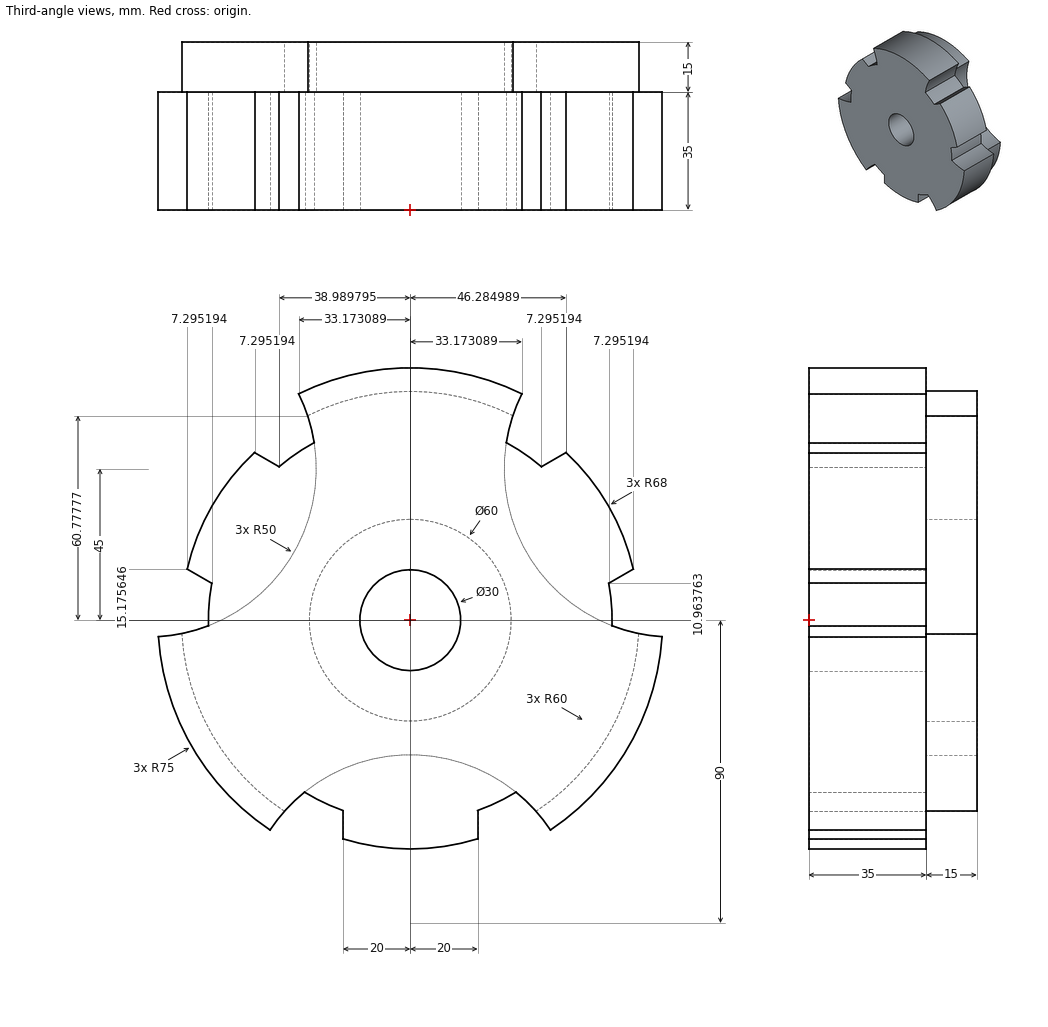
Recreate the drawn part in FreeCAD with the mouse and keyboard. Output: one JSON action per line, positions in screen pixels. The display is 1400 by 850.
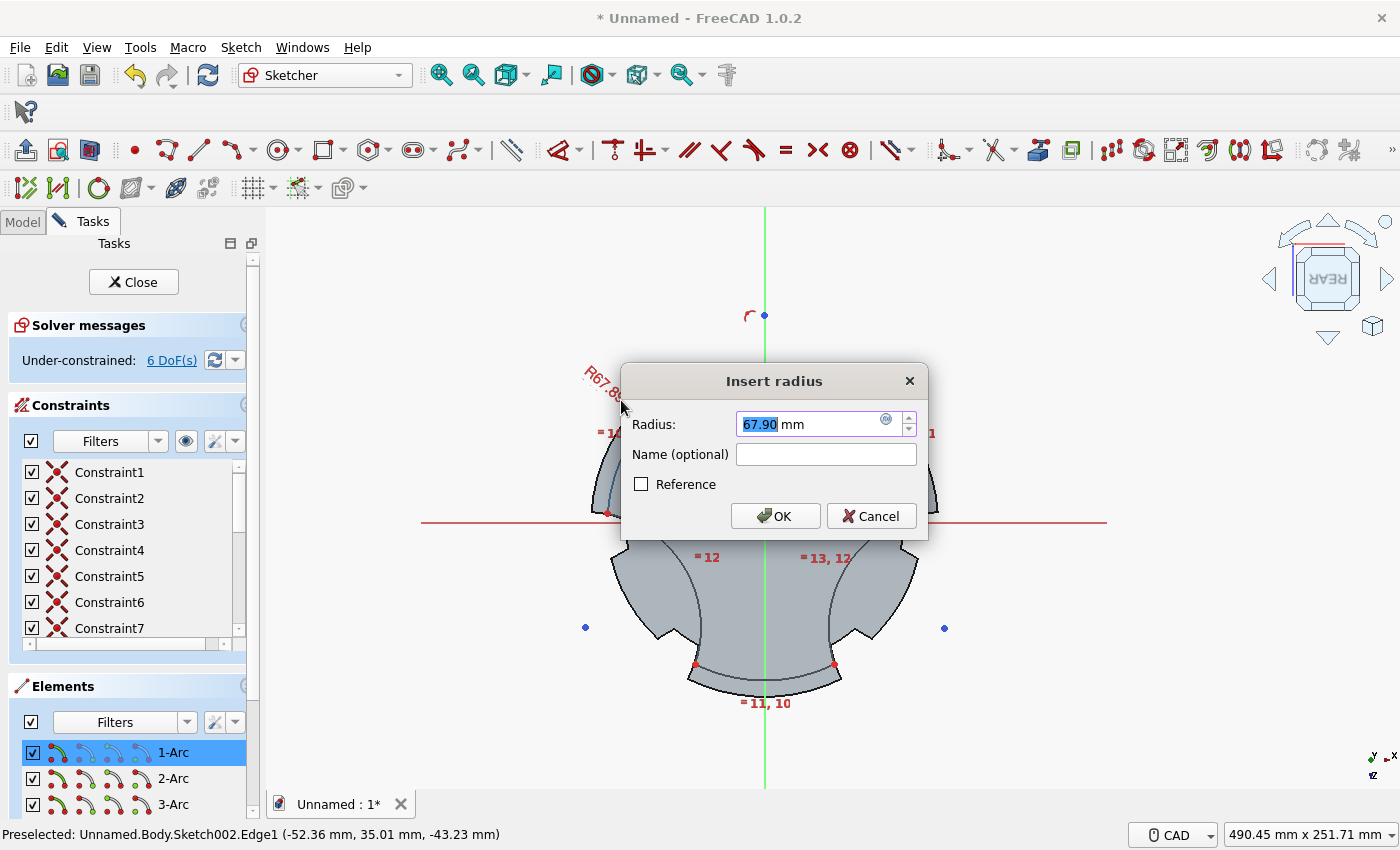
{"action": "type", "text": "68"}
{"action": "key", "text": "Return"}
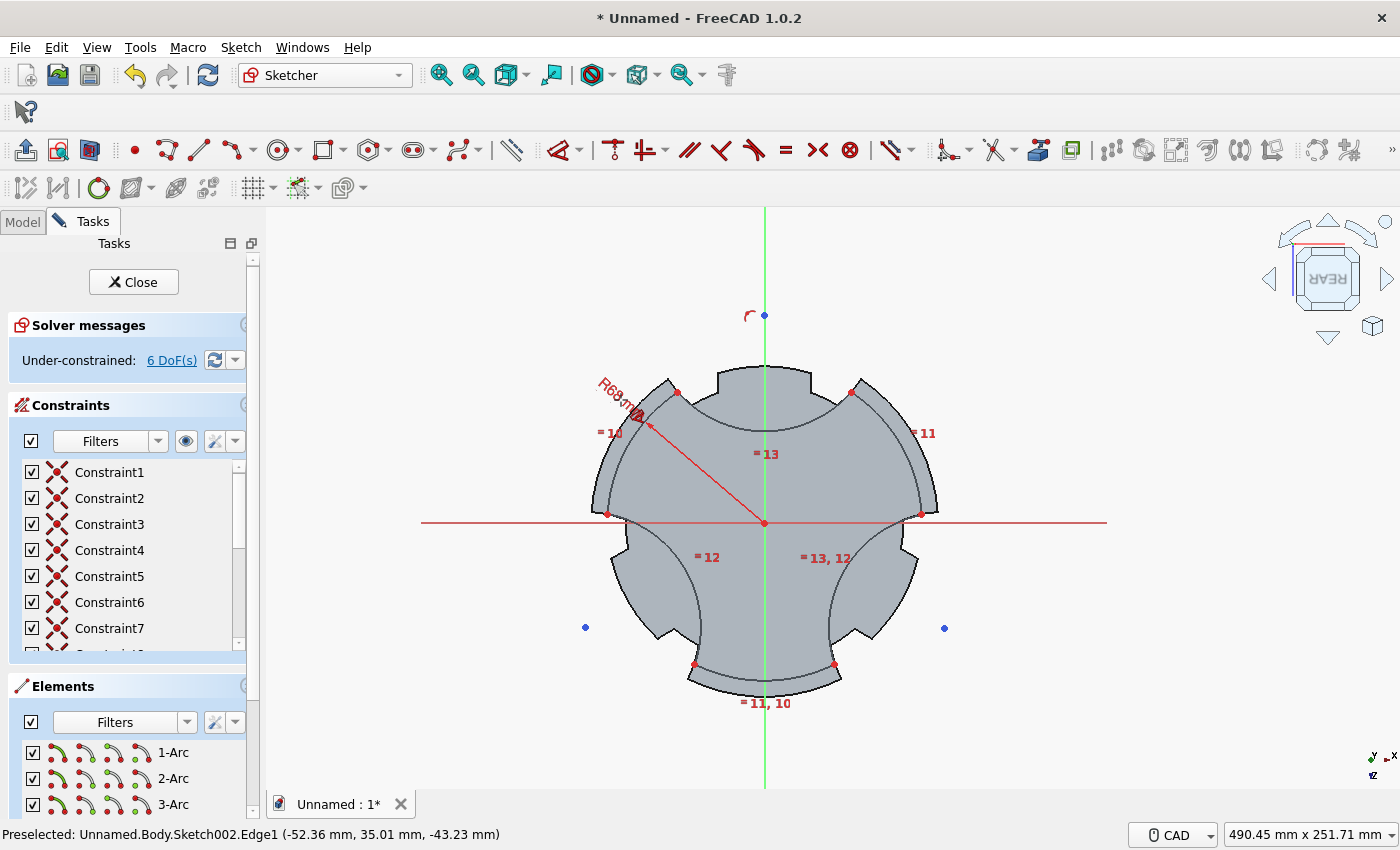
{"action": "left_click", "coordinate": [699, 606]}
{"action": "left_click", "coordinate": [730, 600]}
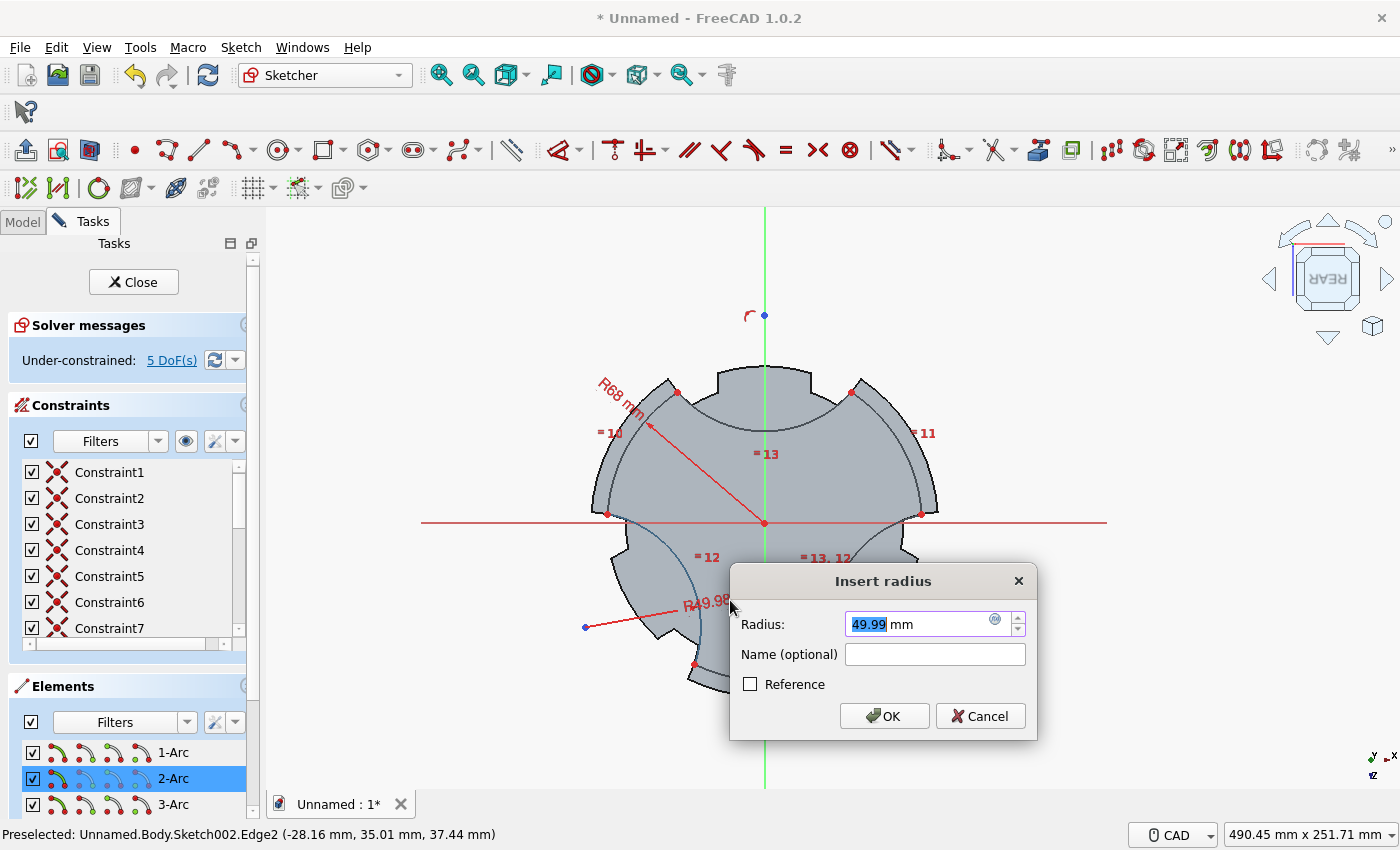
{"action": "type", "text": "50"}
{"action": "key", "text": "Return"}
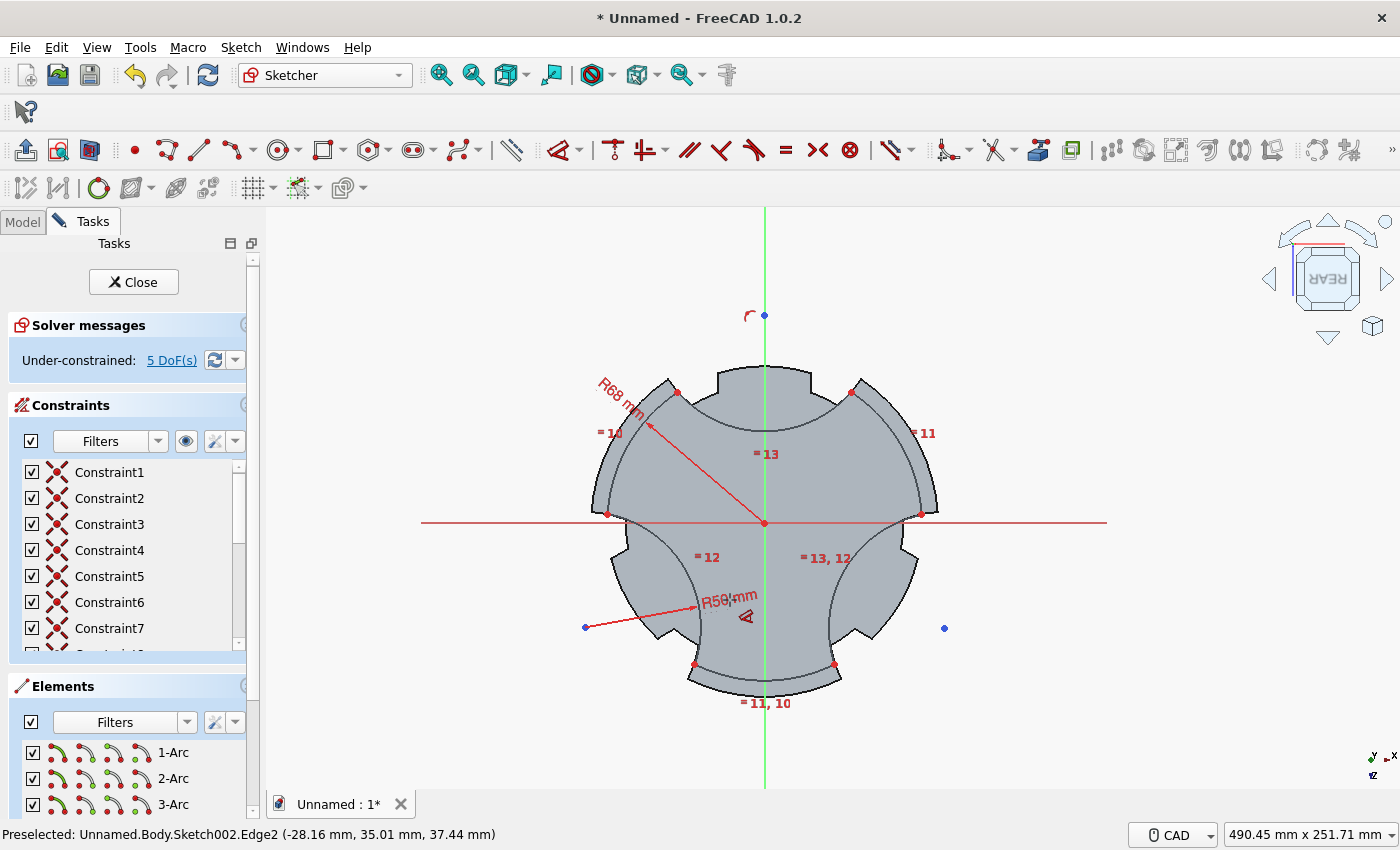
{"action": "left_click", "coordinate": [585, 627]}
{"action": "left_click", "coordinate": [551, 575]}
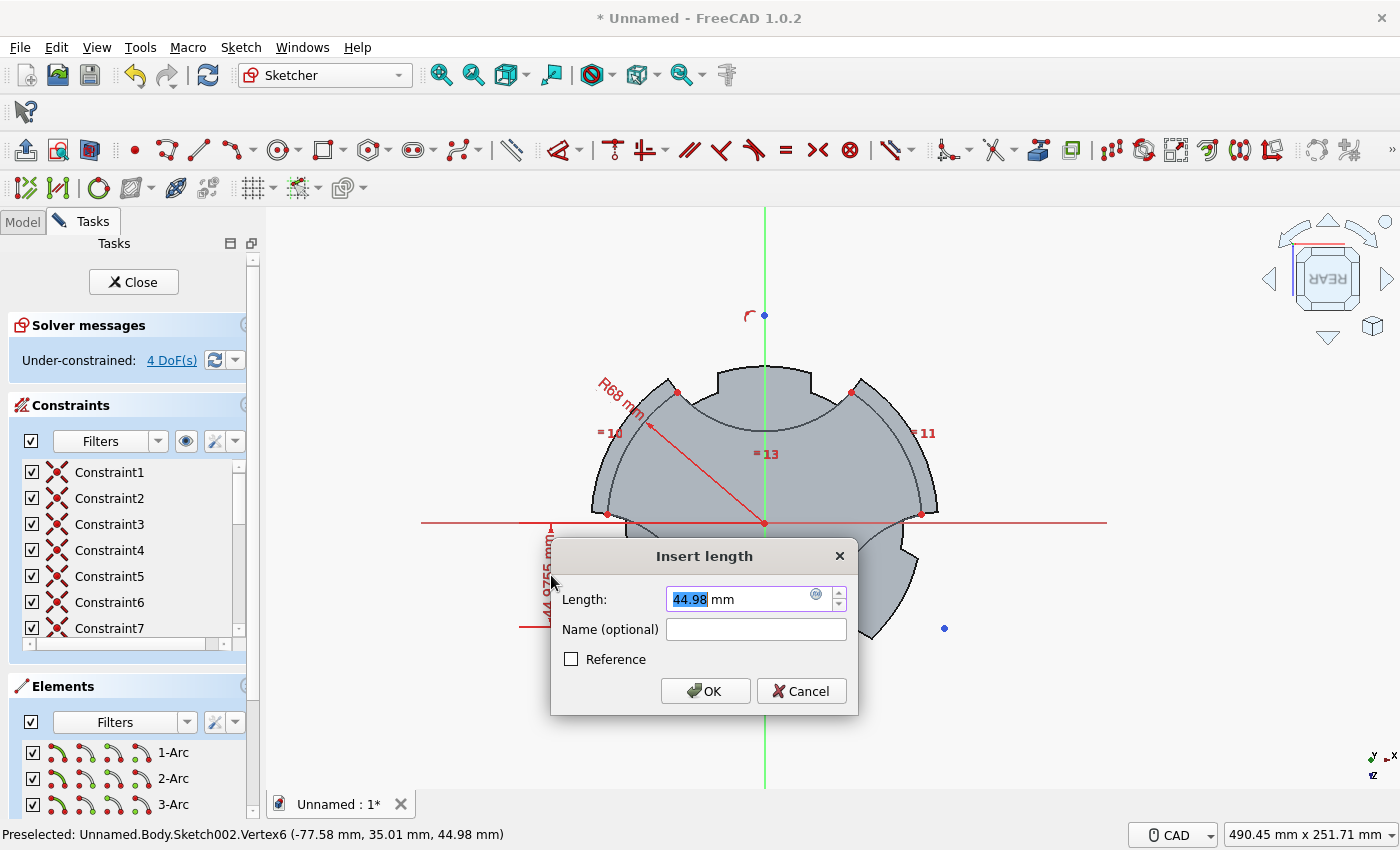
{"action": "type", "text": "45"}
{"action": "key", "text": "Return"}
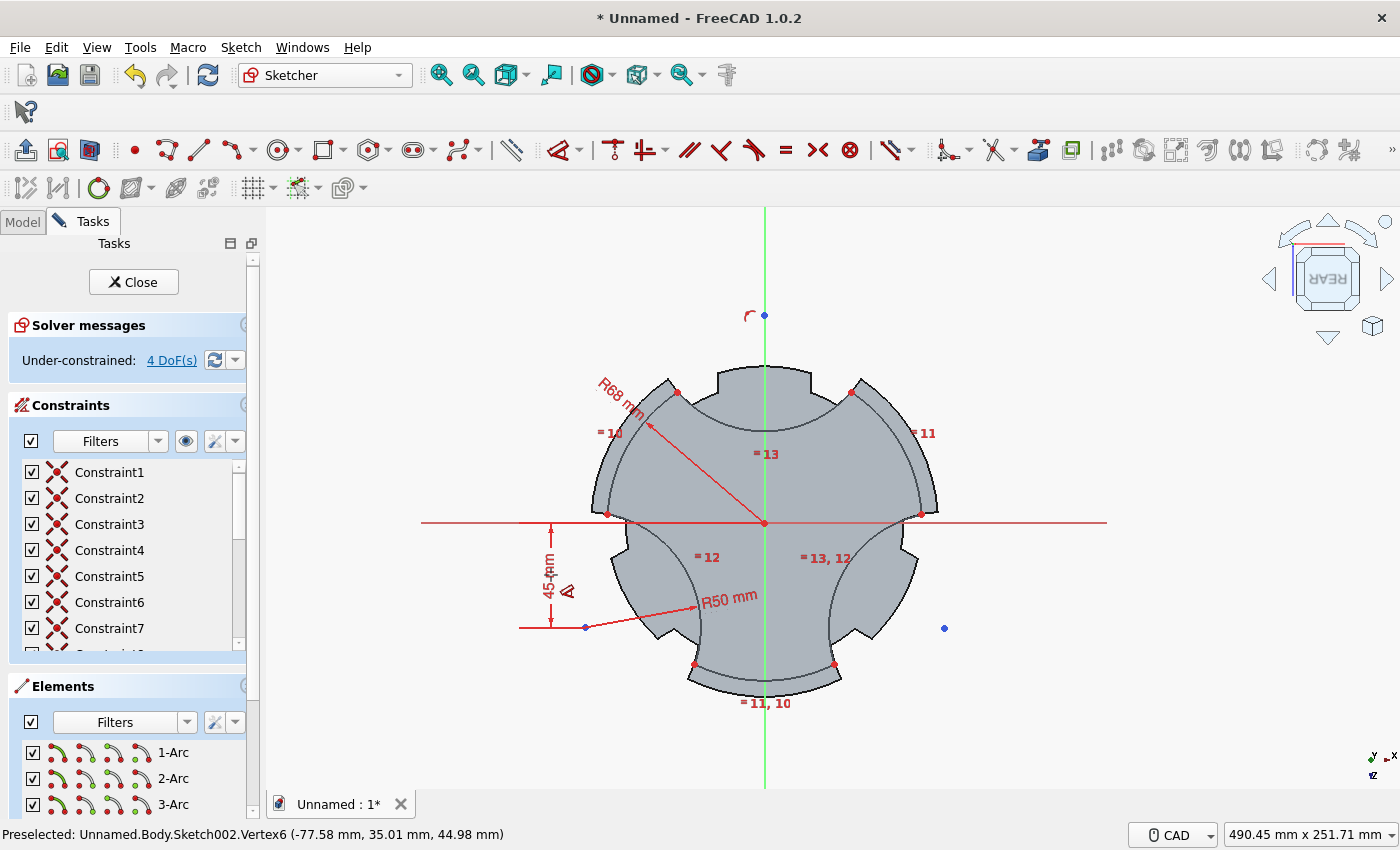
{"action": "left_click", "coordinate": [945, 628]}
{"action": "left_click", "coordinate": [979, 576]}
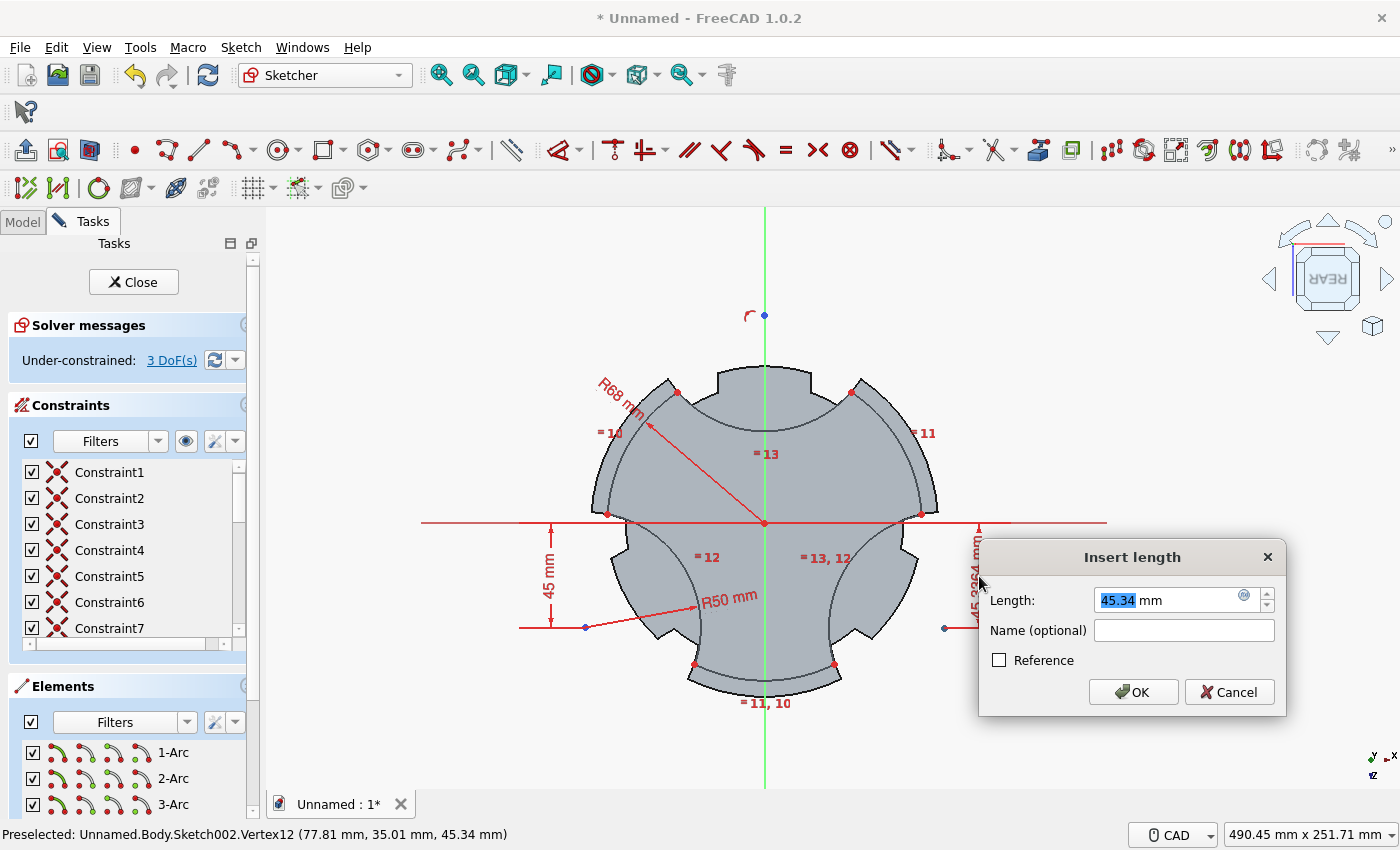
{"action": "type", "text": "45"}
{"action": "key", "text": "Return"}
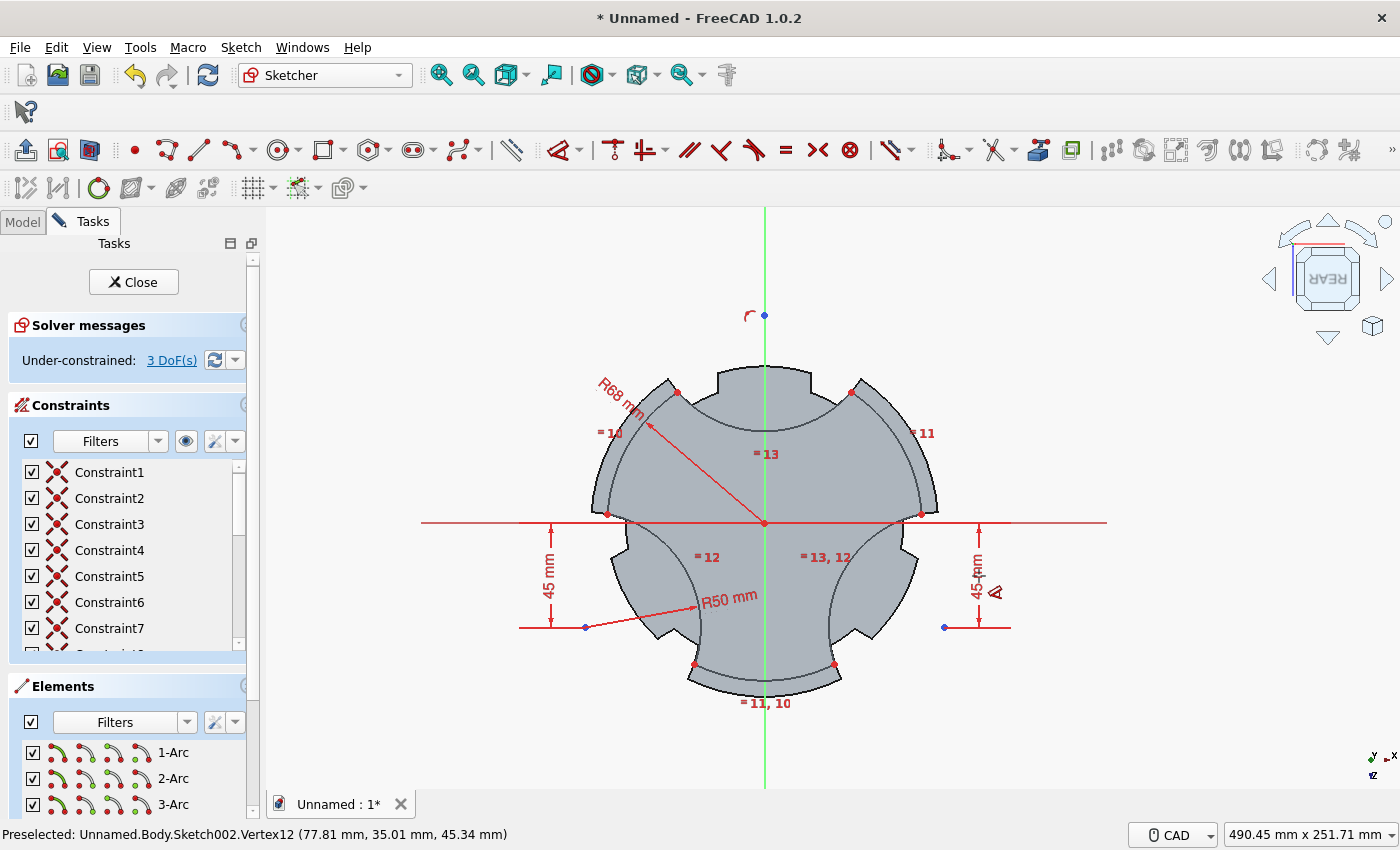
{"action": "left_click", "coordinate": [765, 316]}
{"action": "left_click", "coordinate": [799, 372]}